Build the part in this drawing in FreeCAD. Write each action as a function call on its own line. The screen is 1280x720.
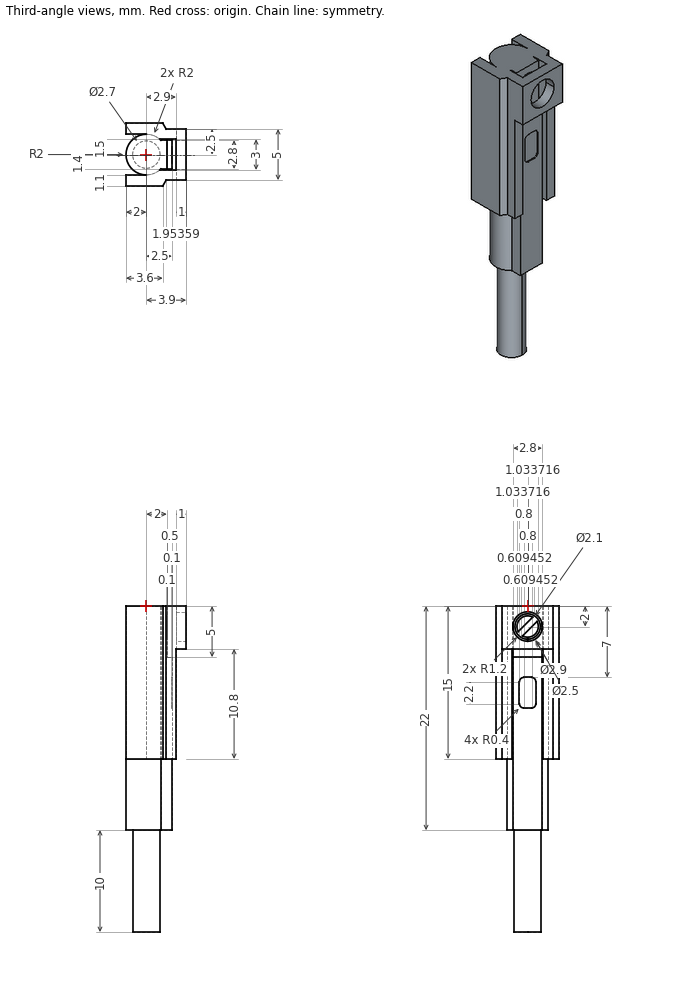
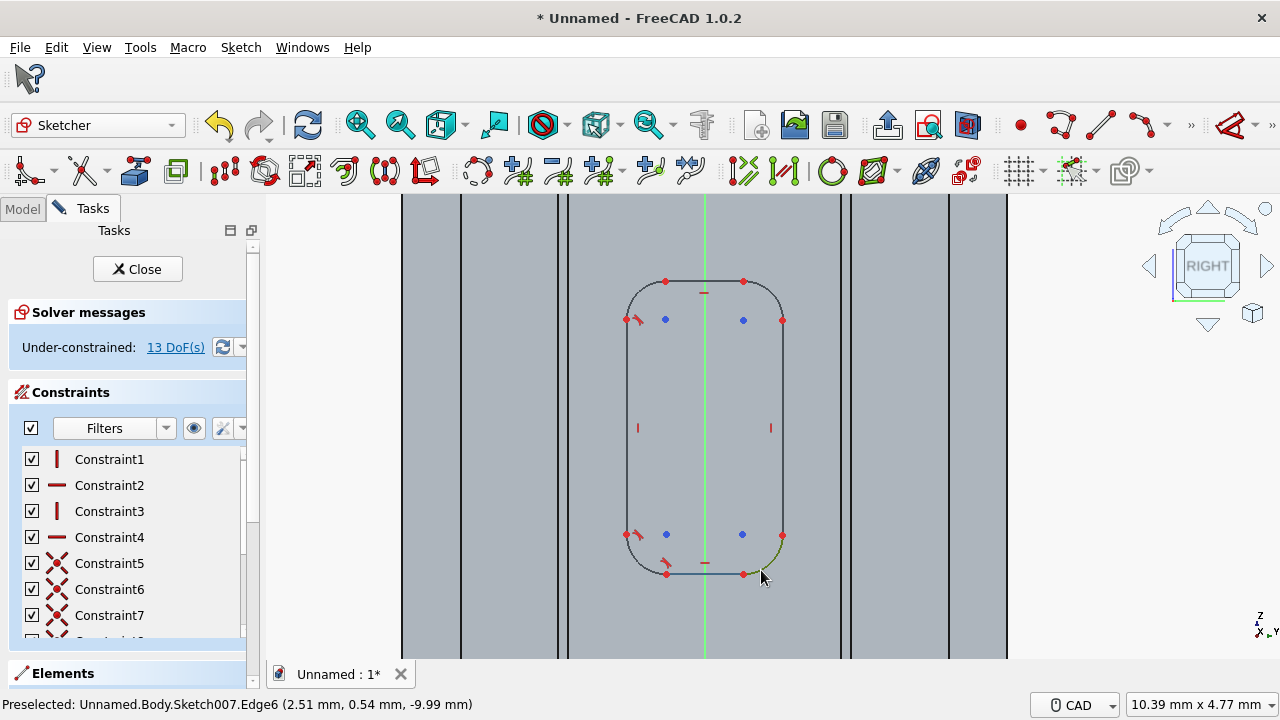
key(t)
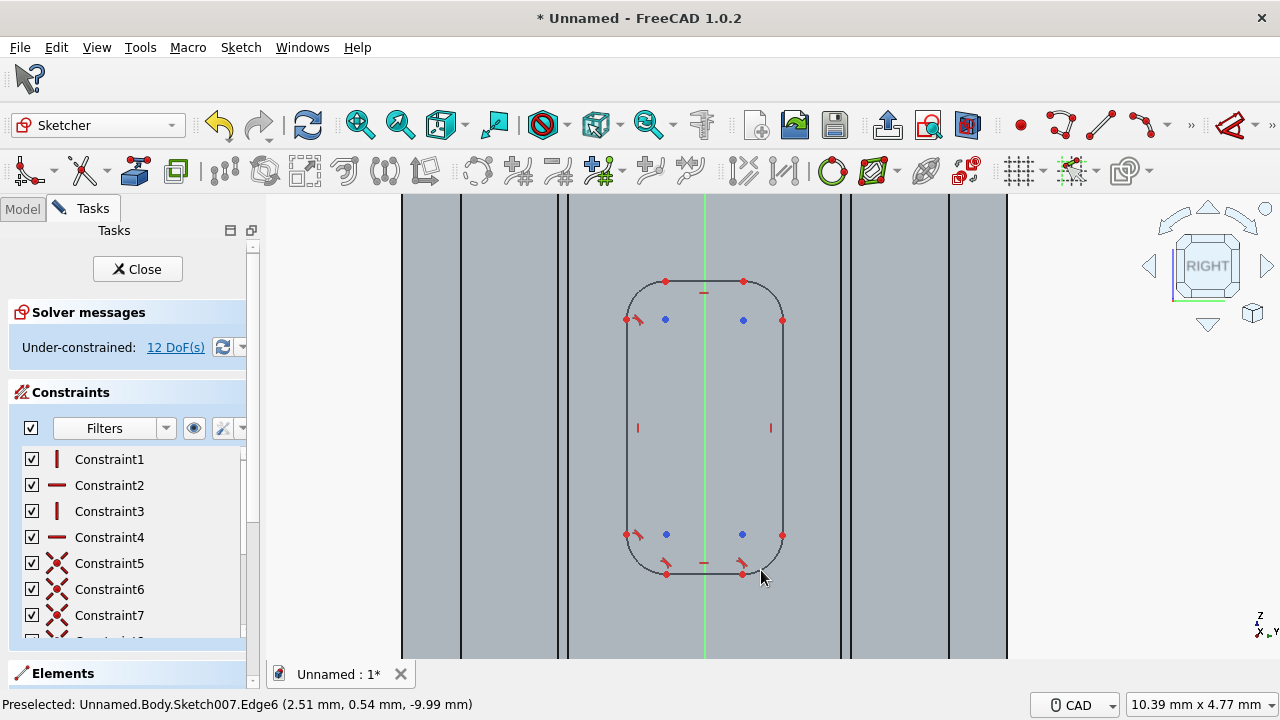
click(783, 471)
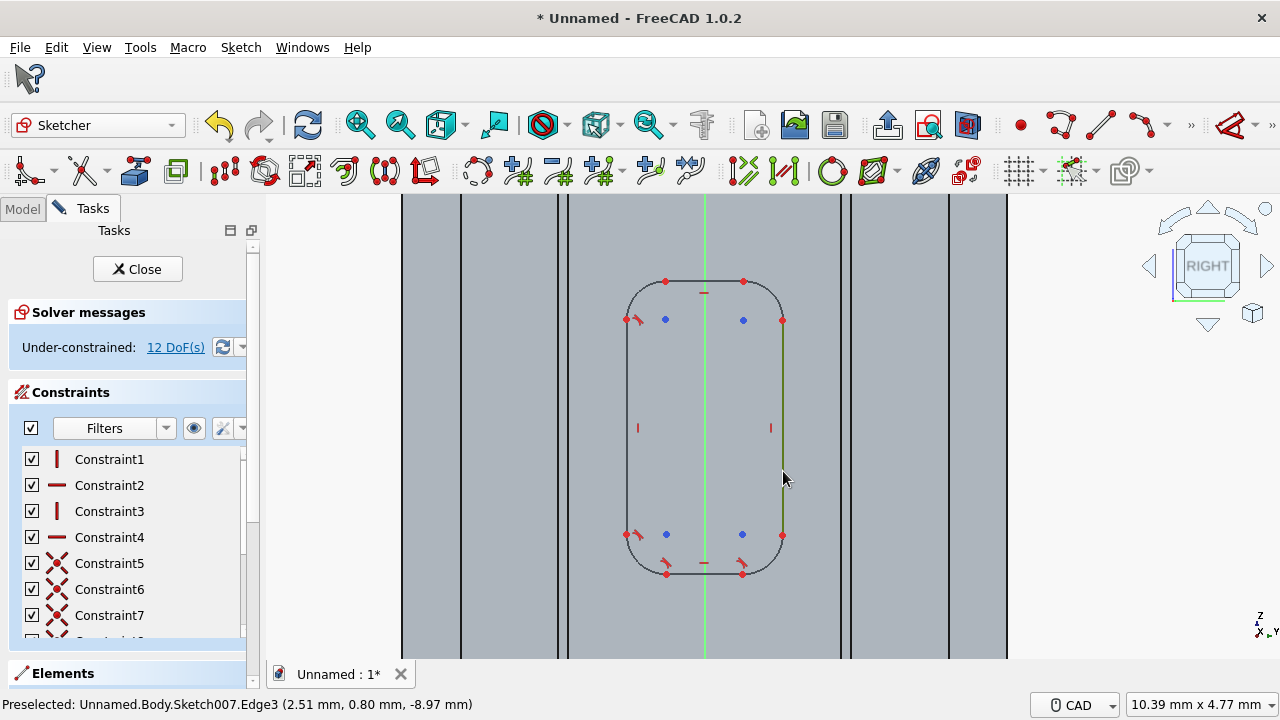
click(761, 570)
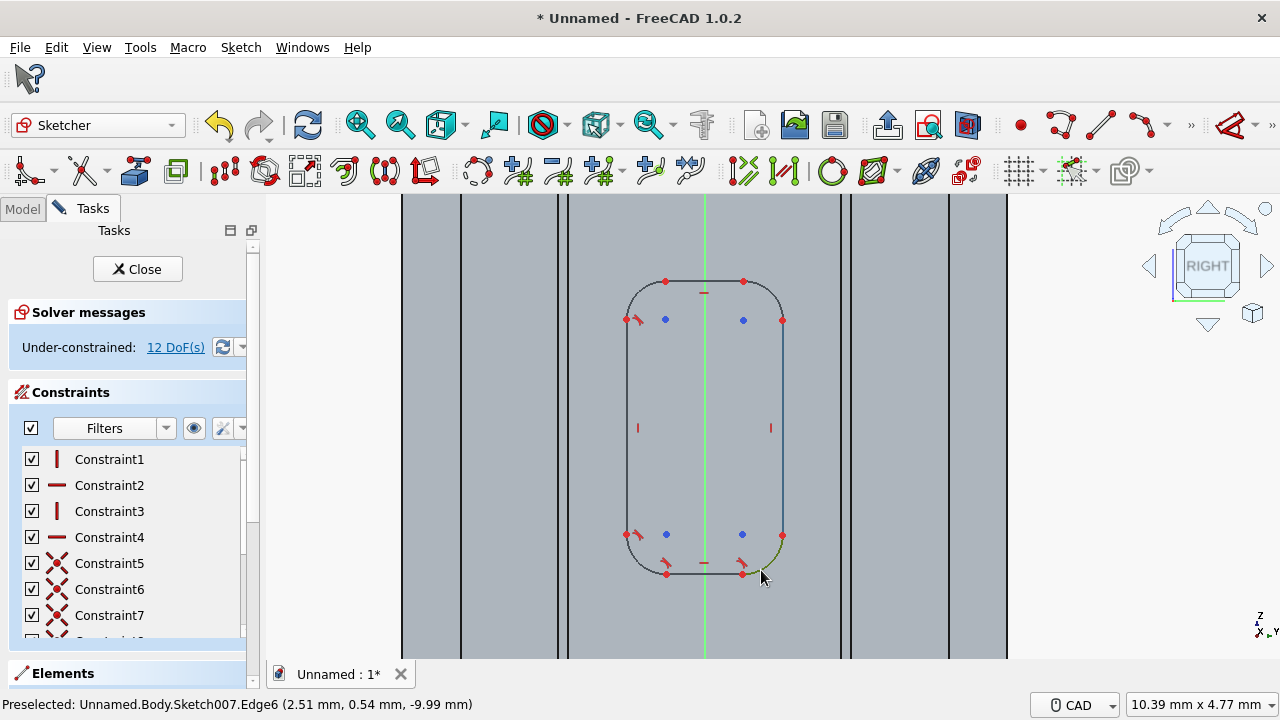
key(t)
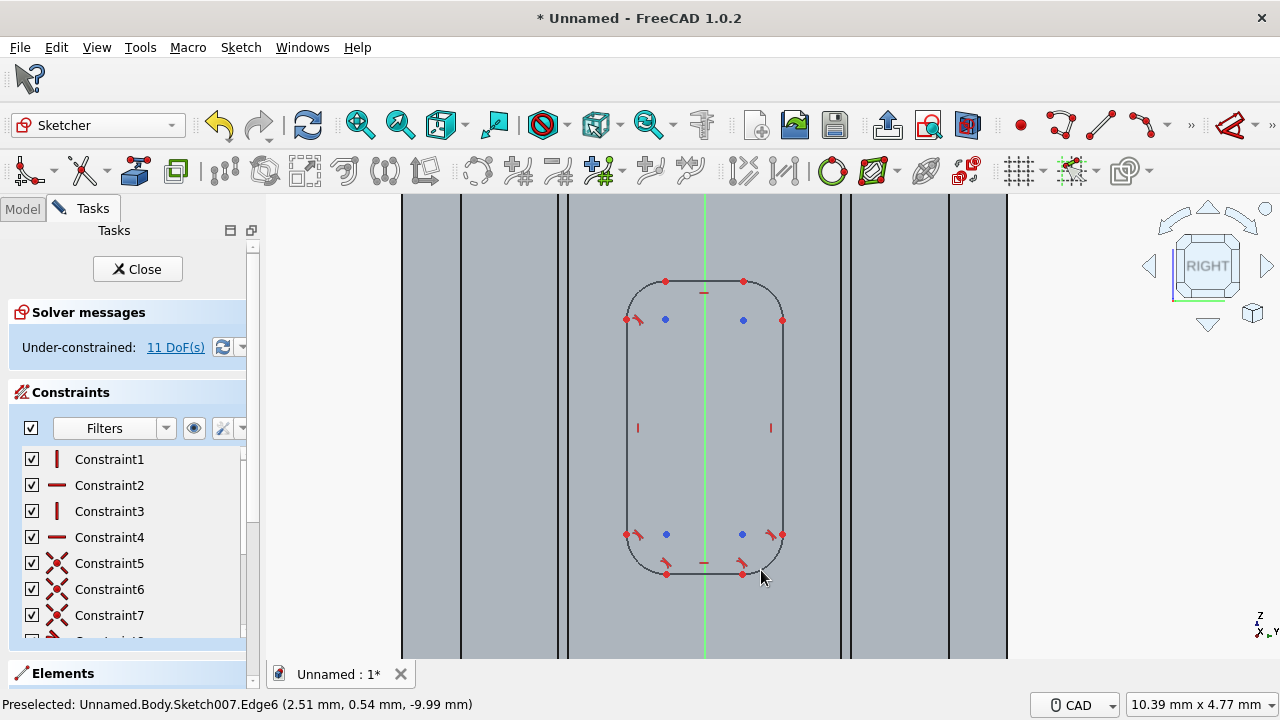
click(783, 470)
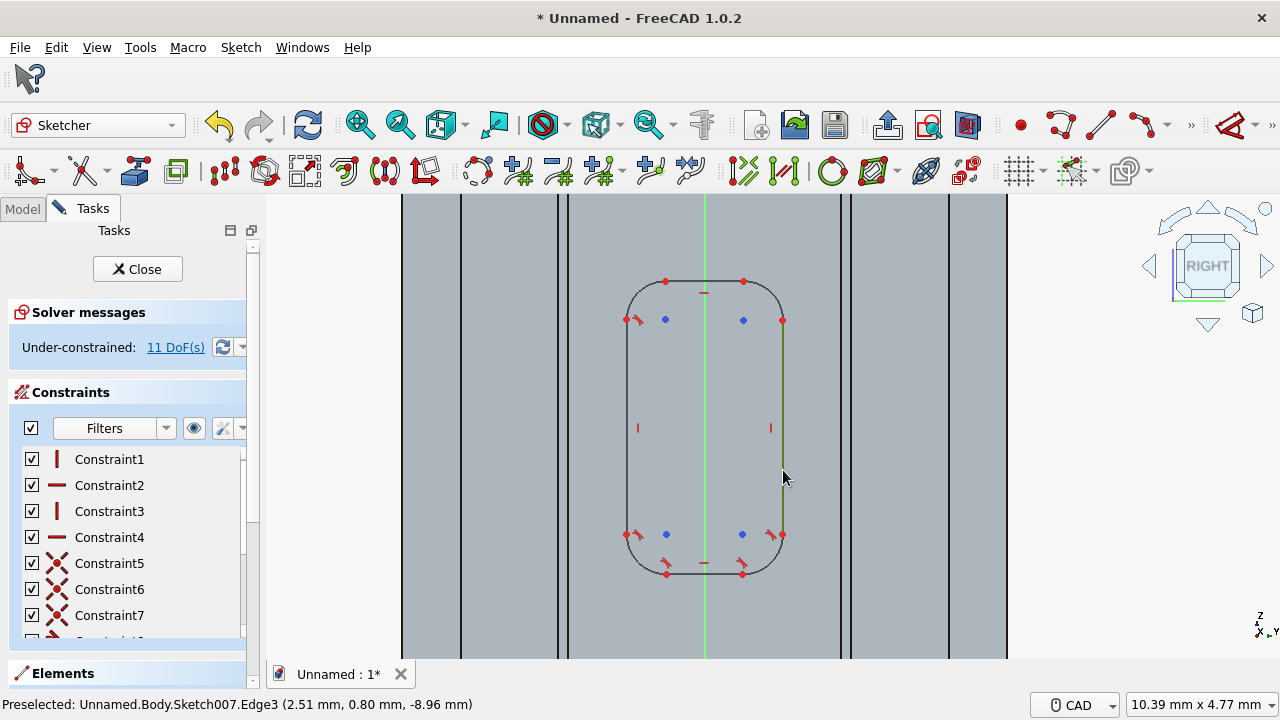
click(779, 303)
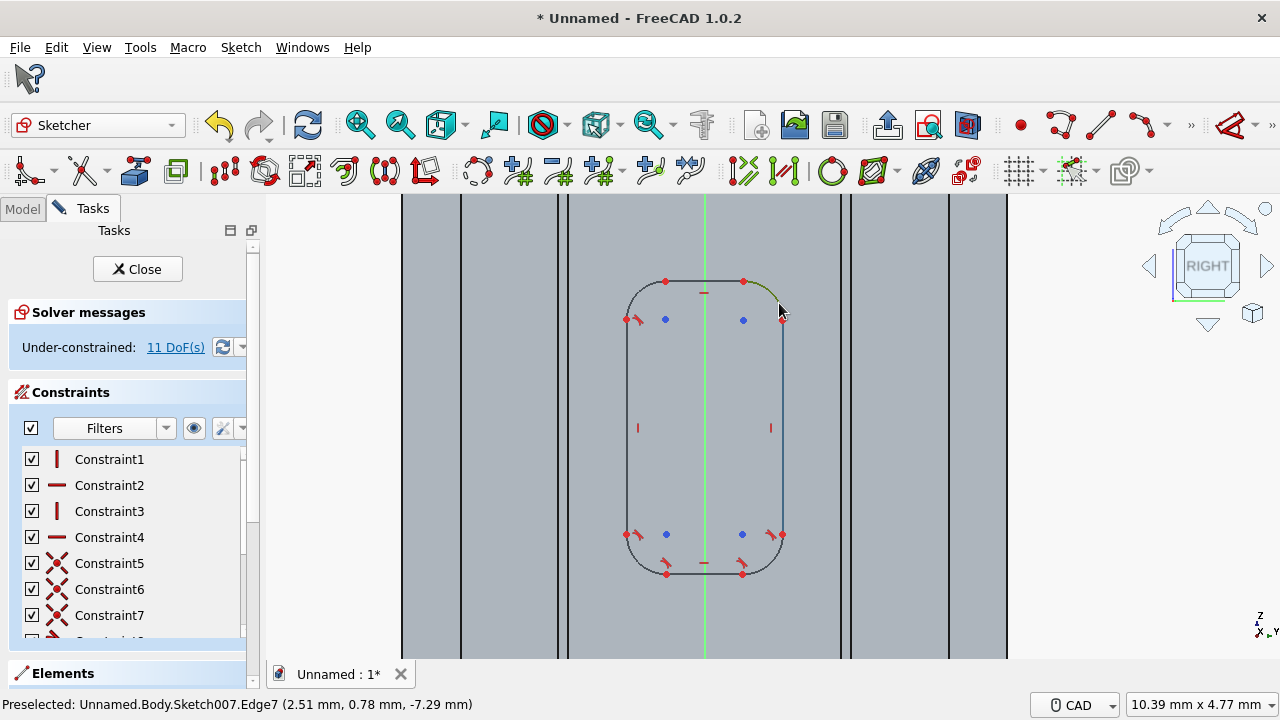
key(t)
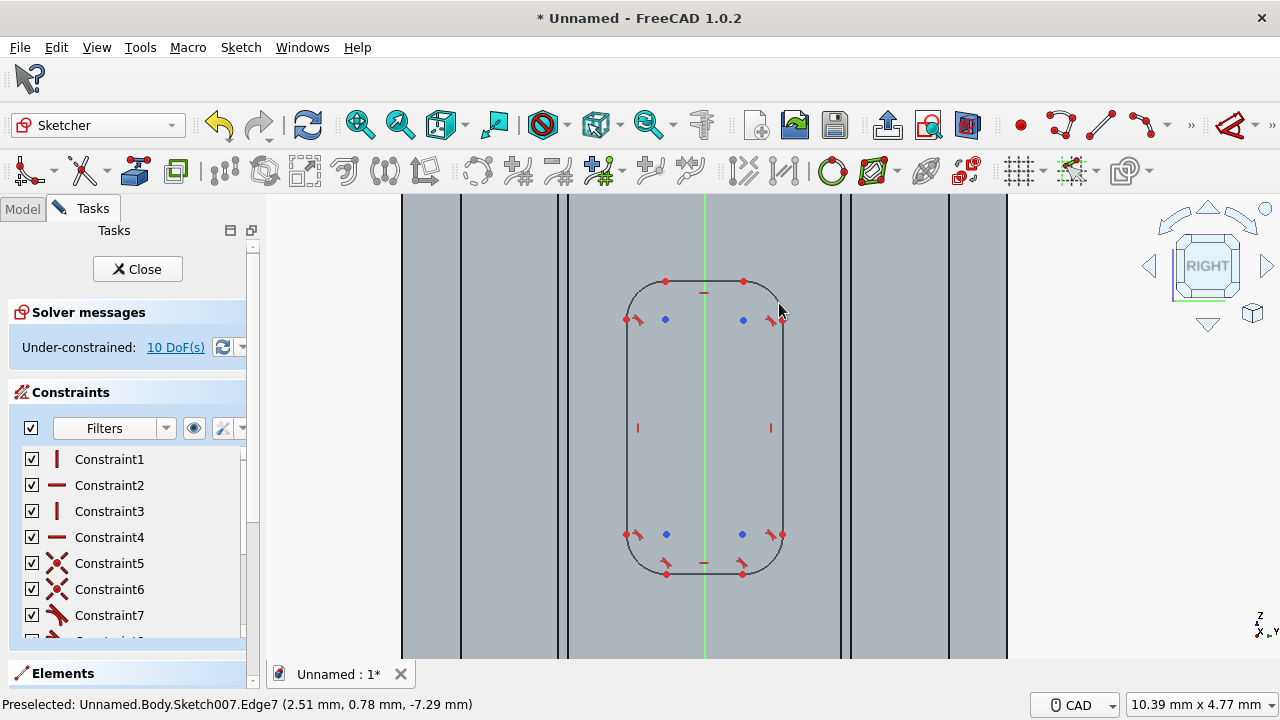
click(721, 281)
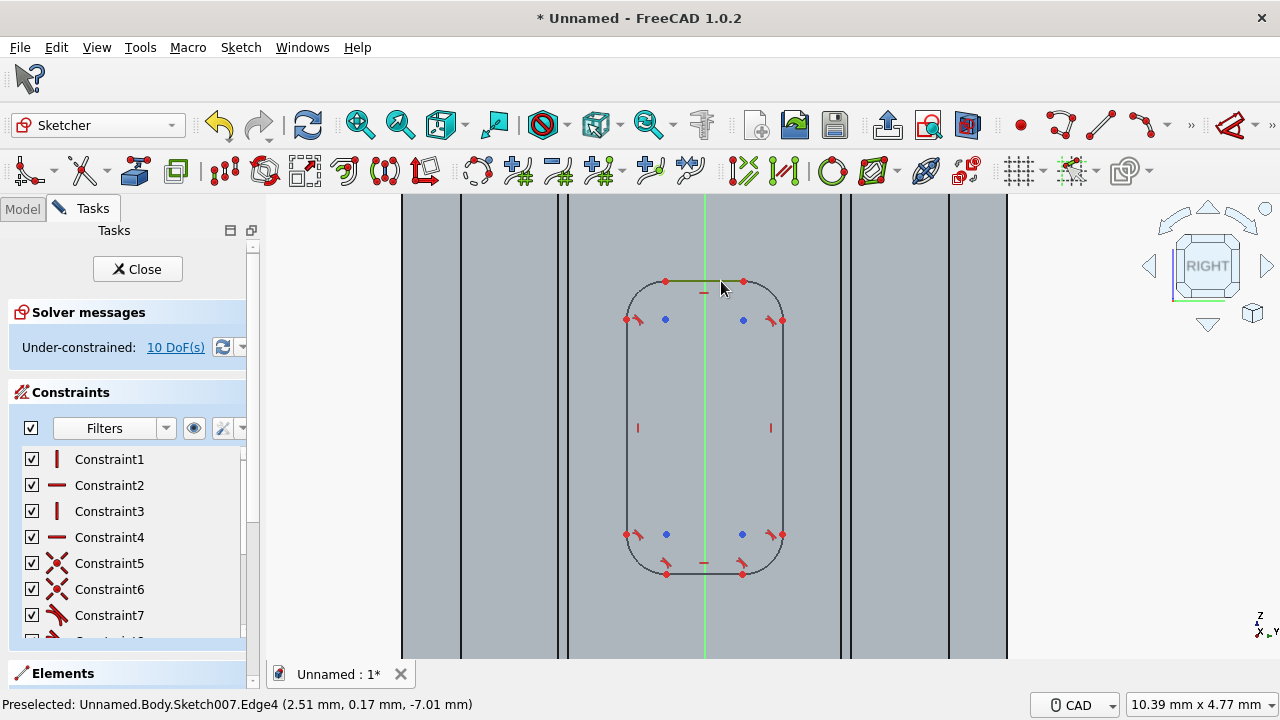
click(779, 303)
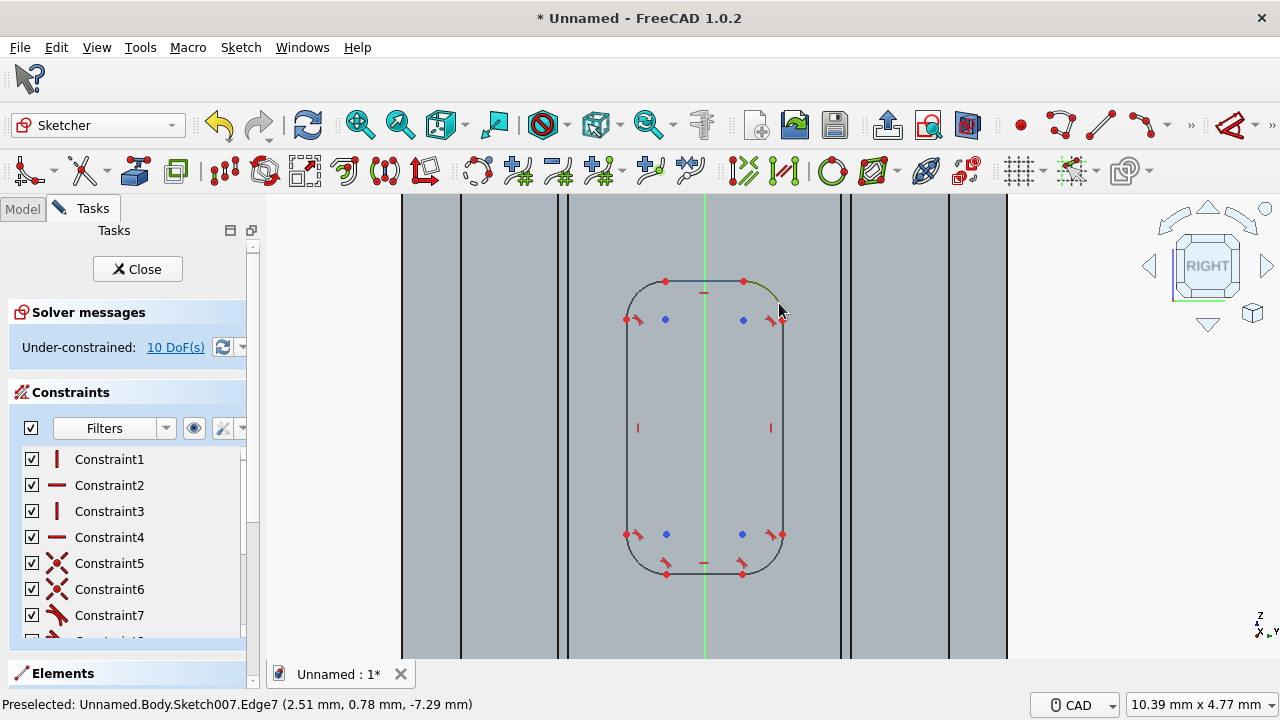
key(t)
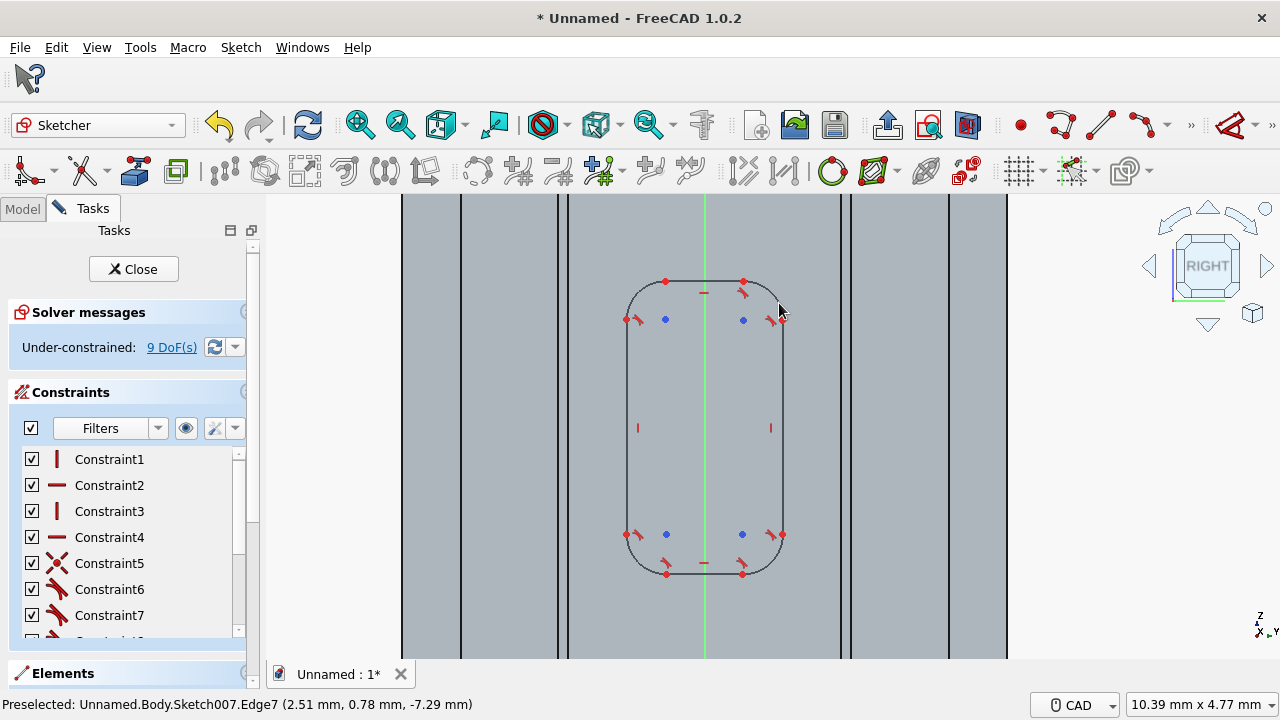
click(721, 281)